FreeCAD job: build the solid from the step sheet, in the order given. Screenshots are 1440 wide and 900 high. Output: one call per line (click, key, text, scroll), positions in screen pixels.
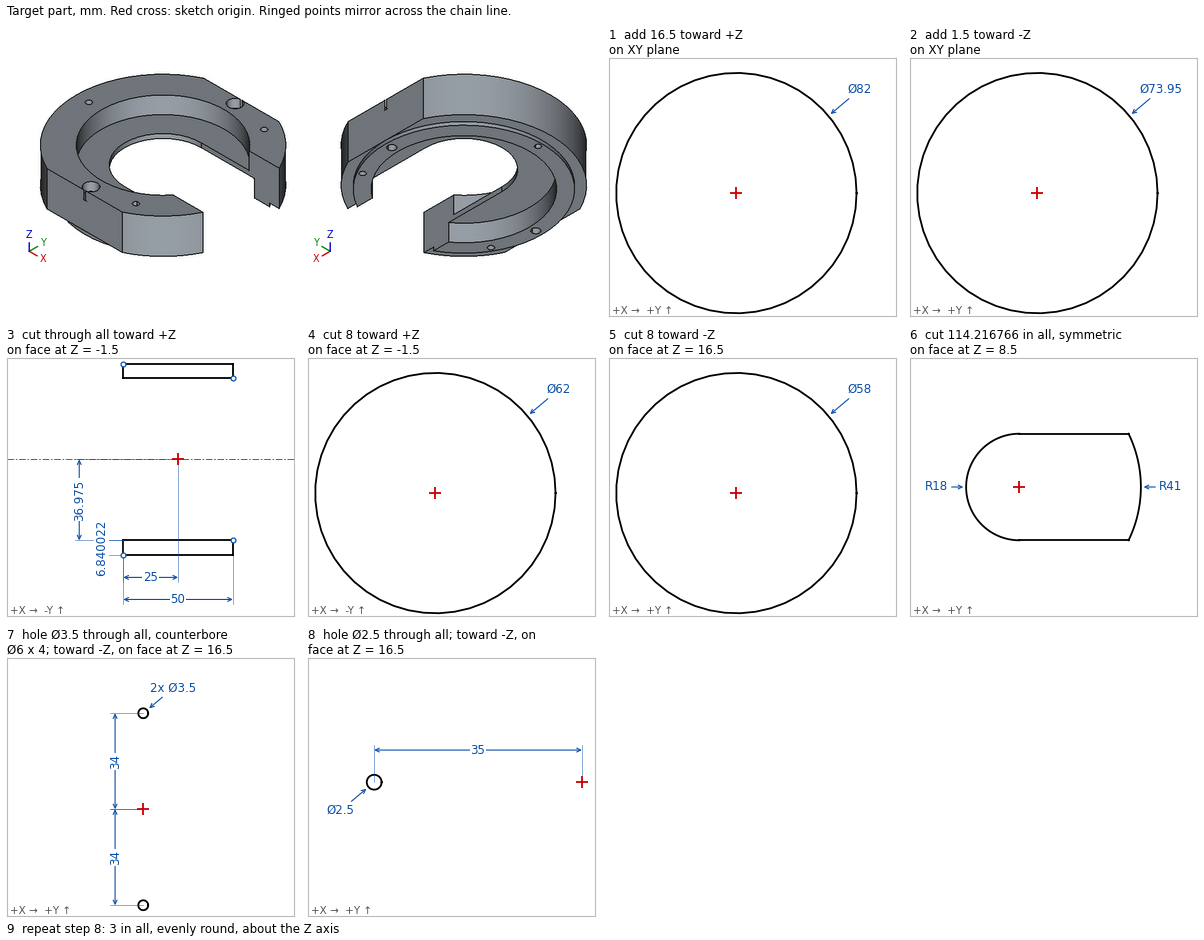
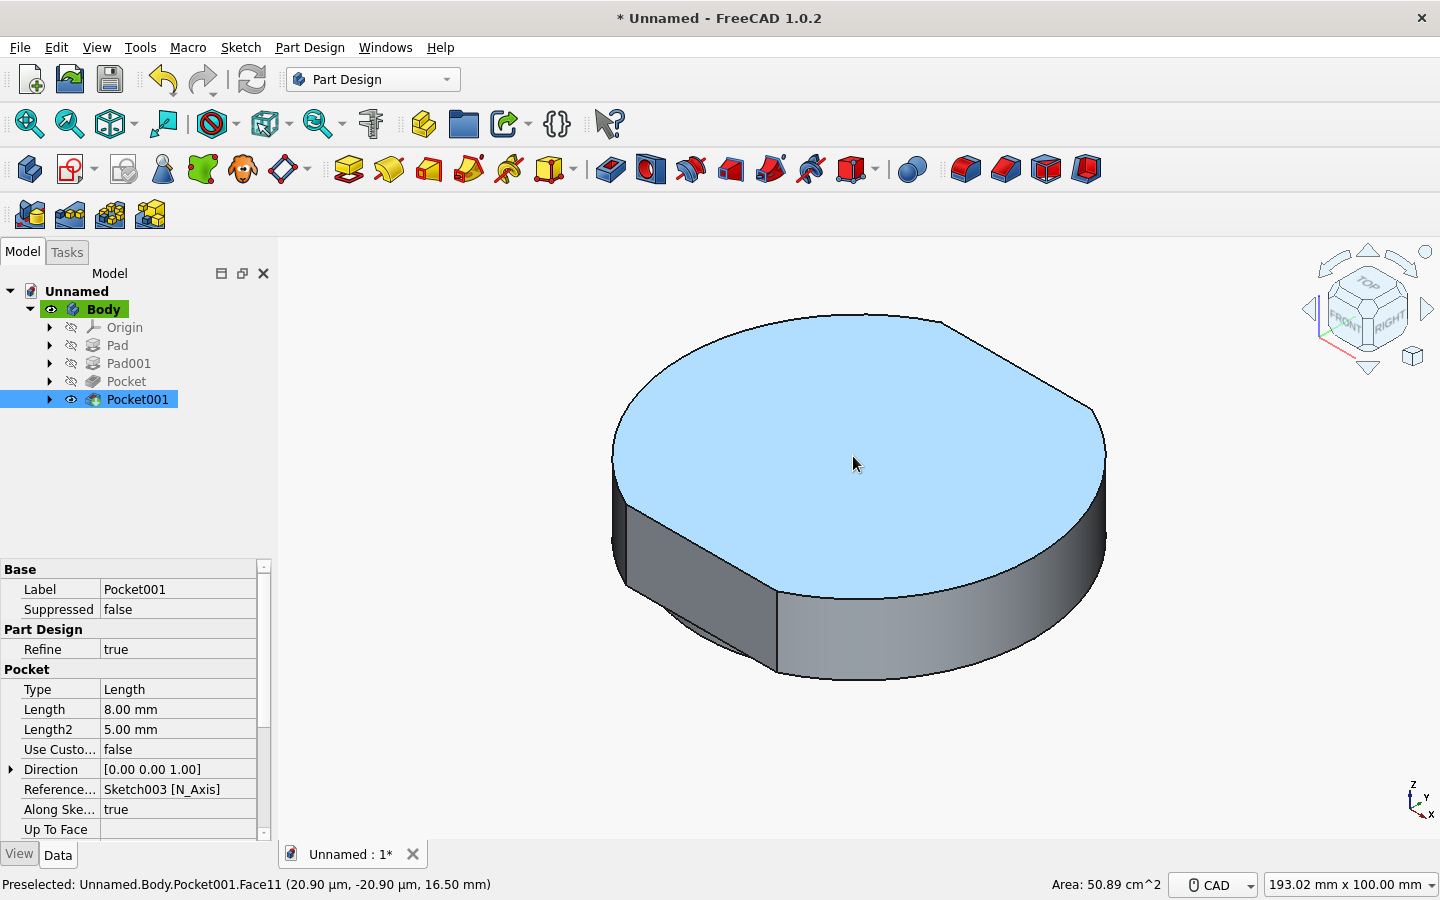
click(70, 170)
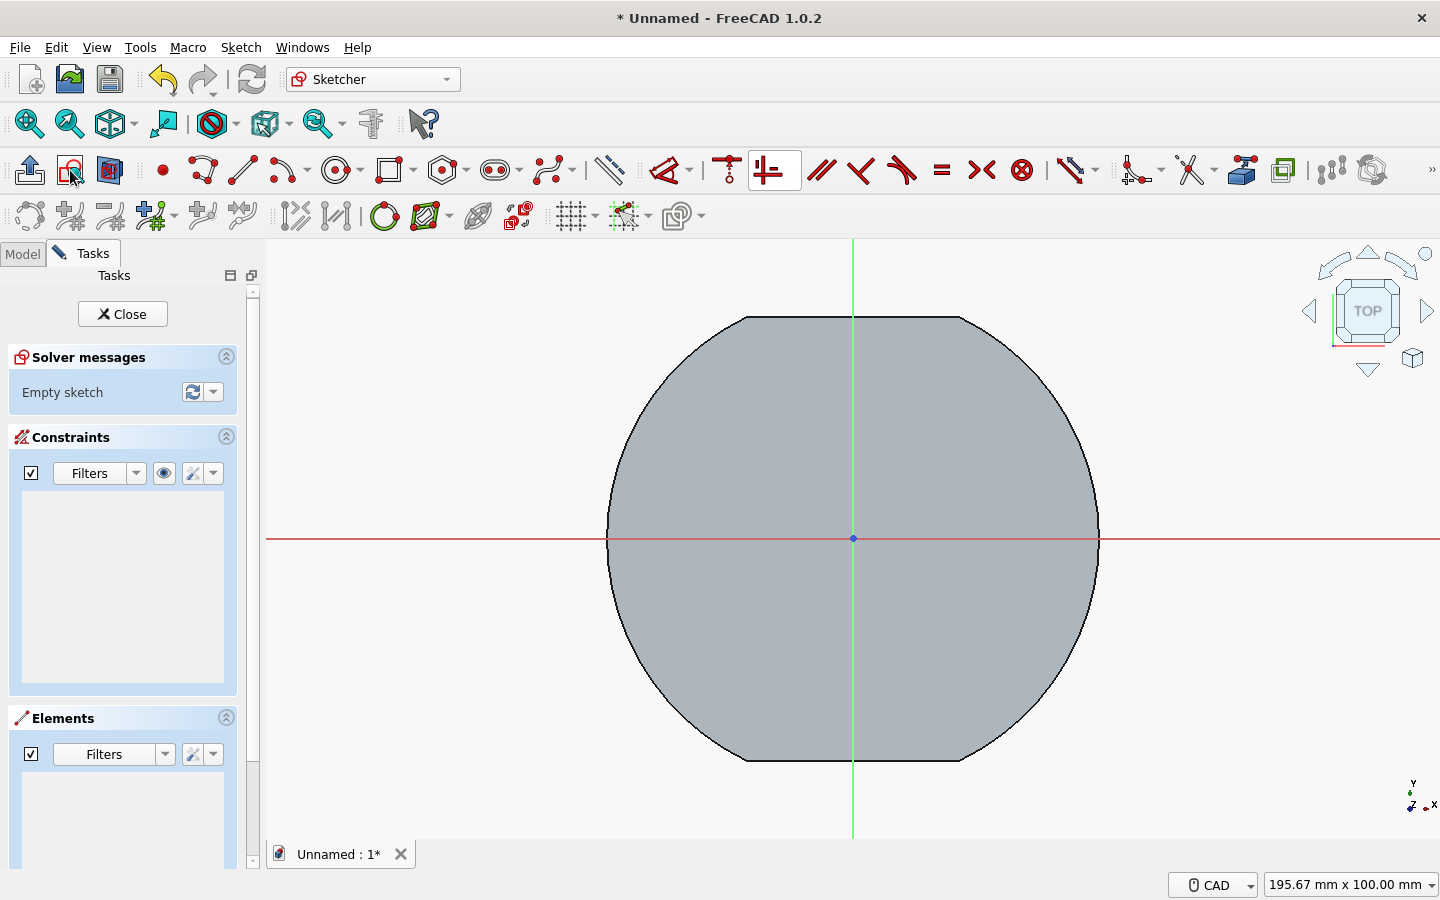
click(336, 170)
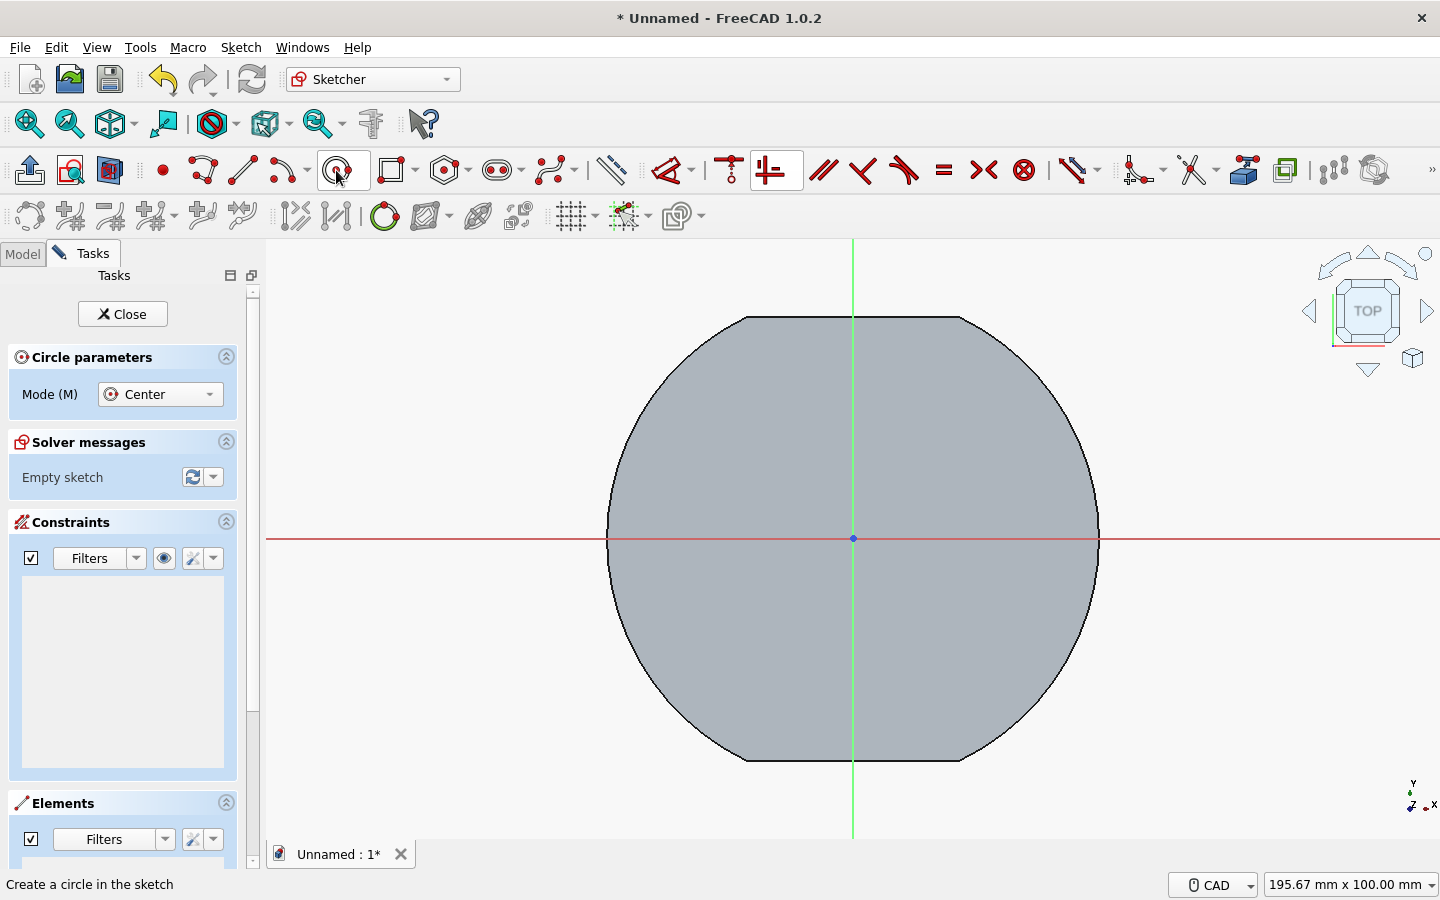
click(853, 539)
click(976, 416)
key(Escape)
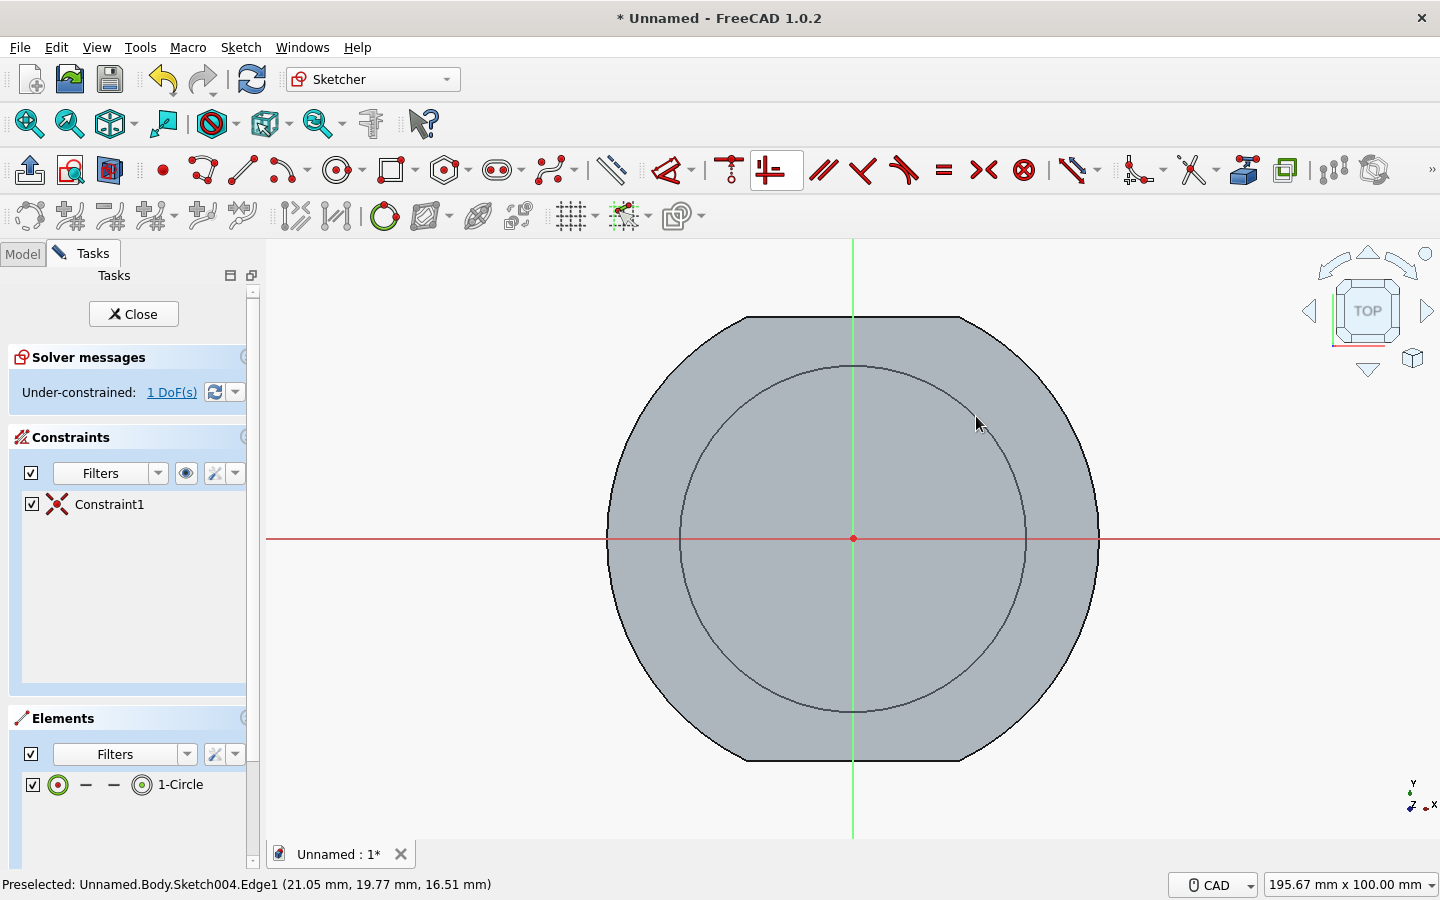
key(d)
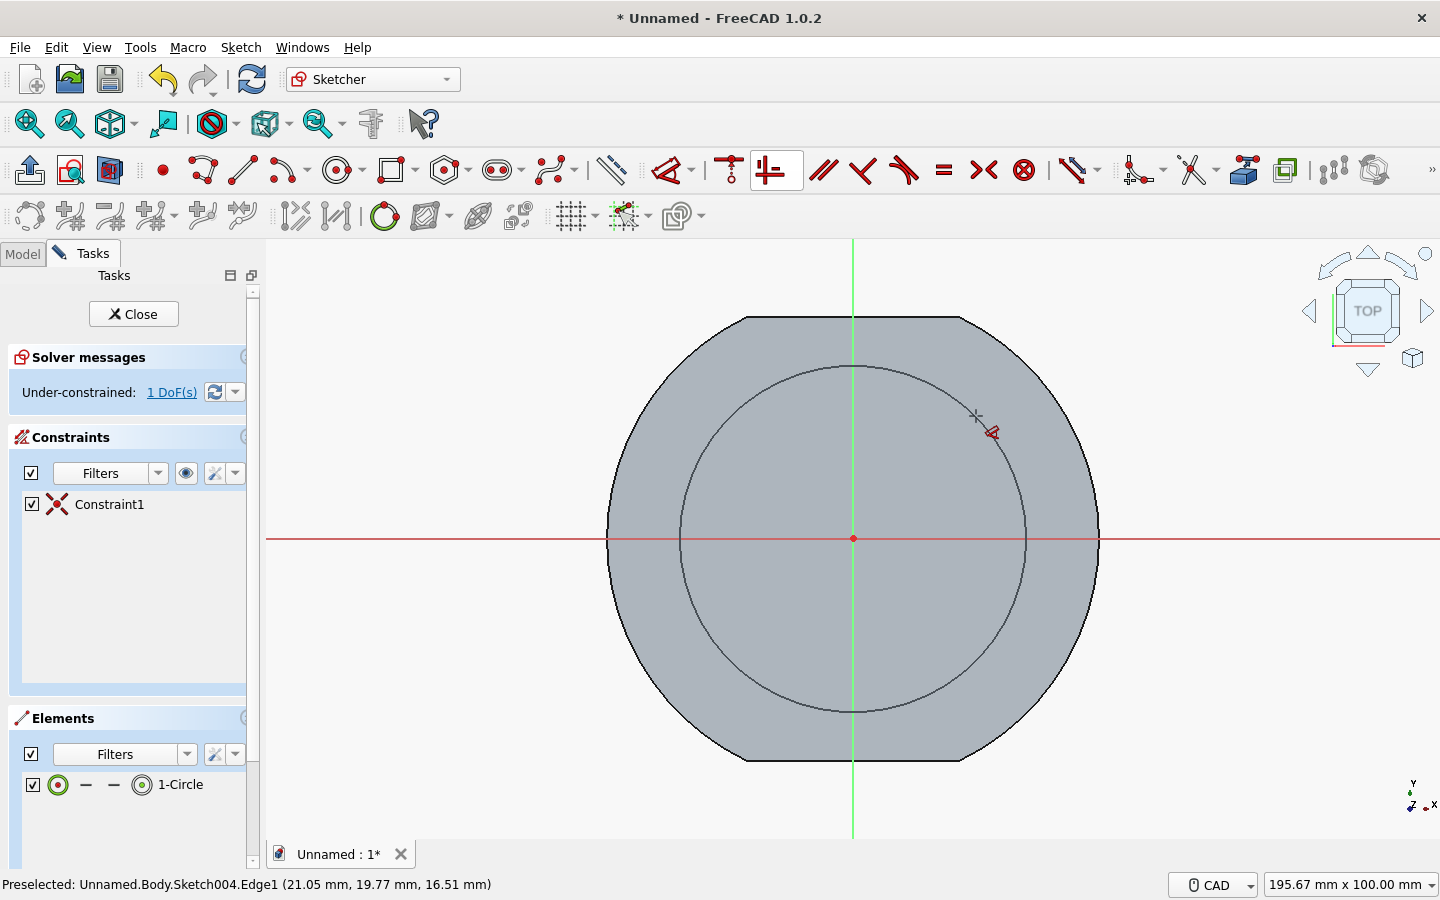
click(975, 416)
click(998, 393)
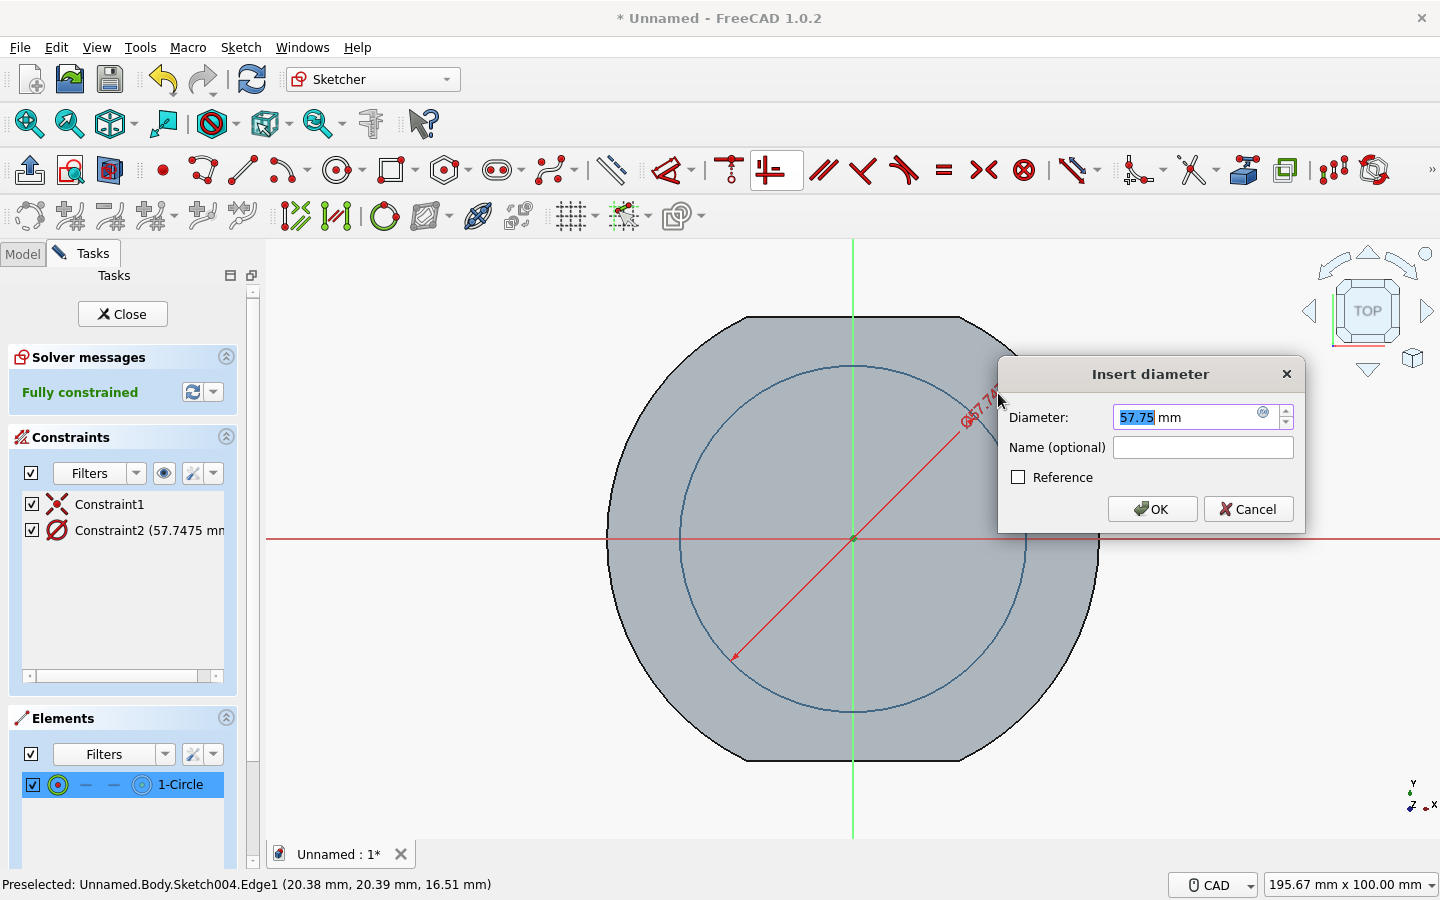
text(58)
key(Return)
key(Escape)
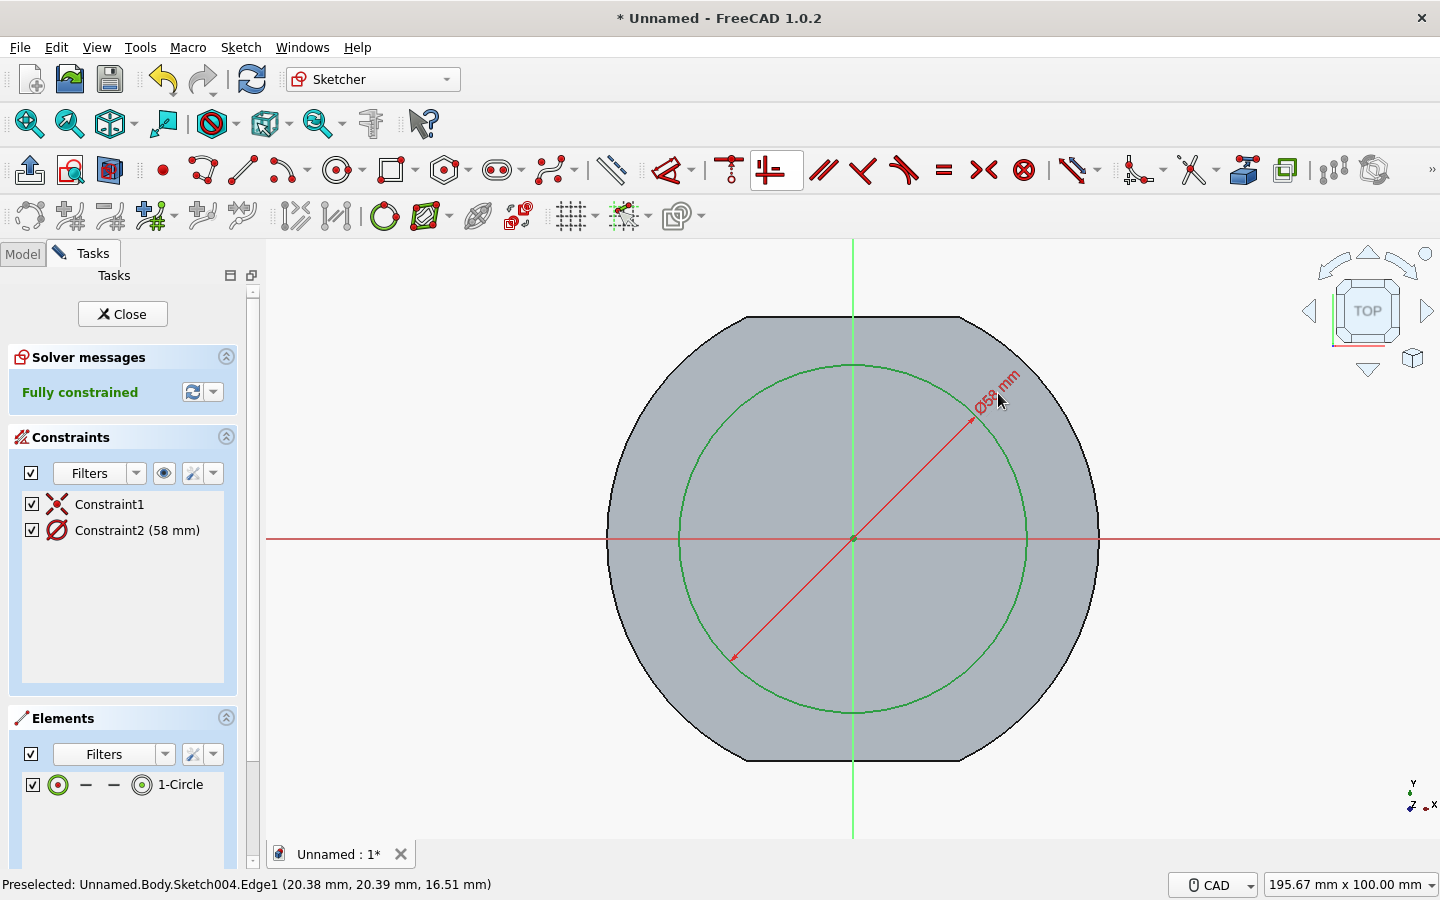
click(123, 314)